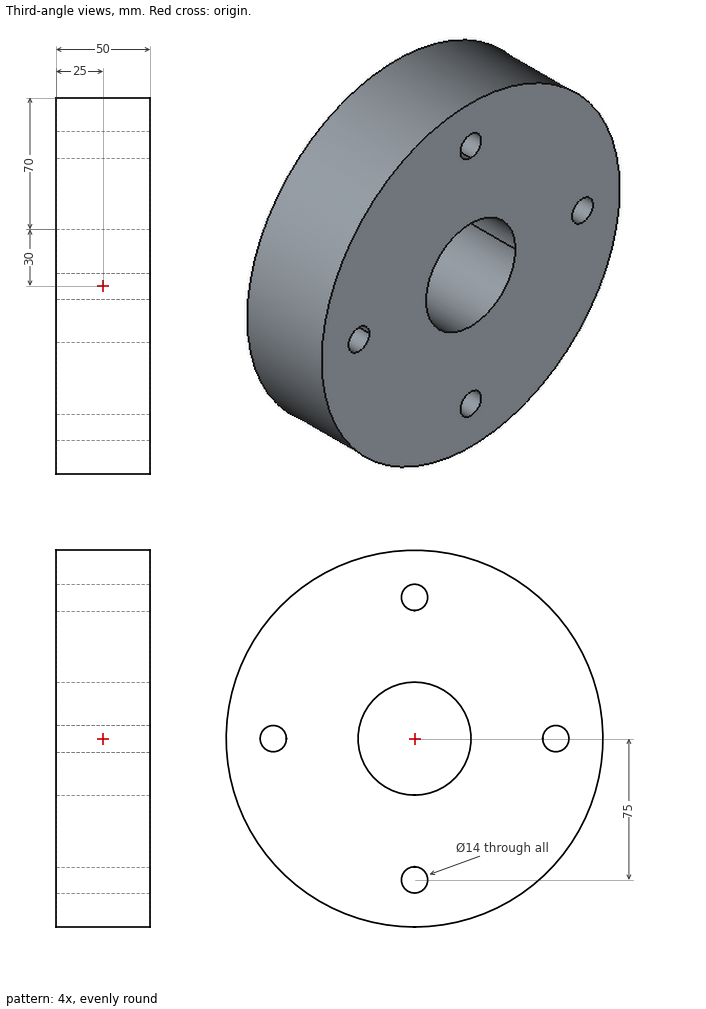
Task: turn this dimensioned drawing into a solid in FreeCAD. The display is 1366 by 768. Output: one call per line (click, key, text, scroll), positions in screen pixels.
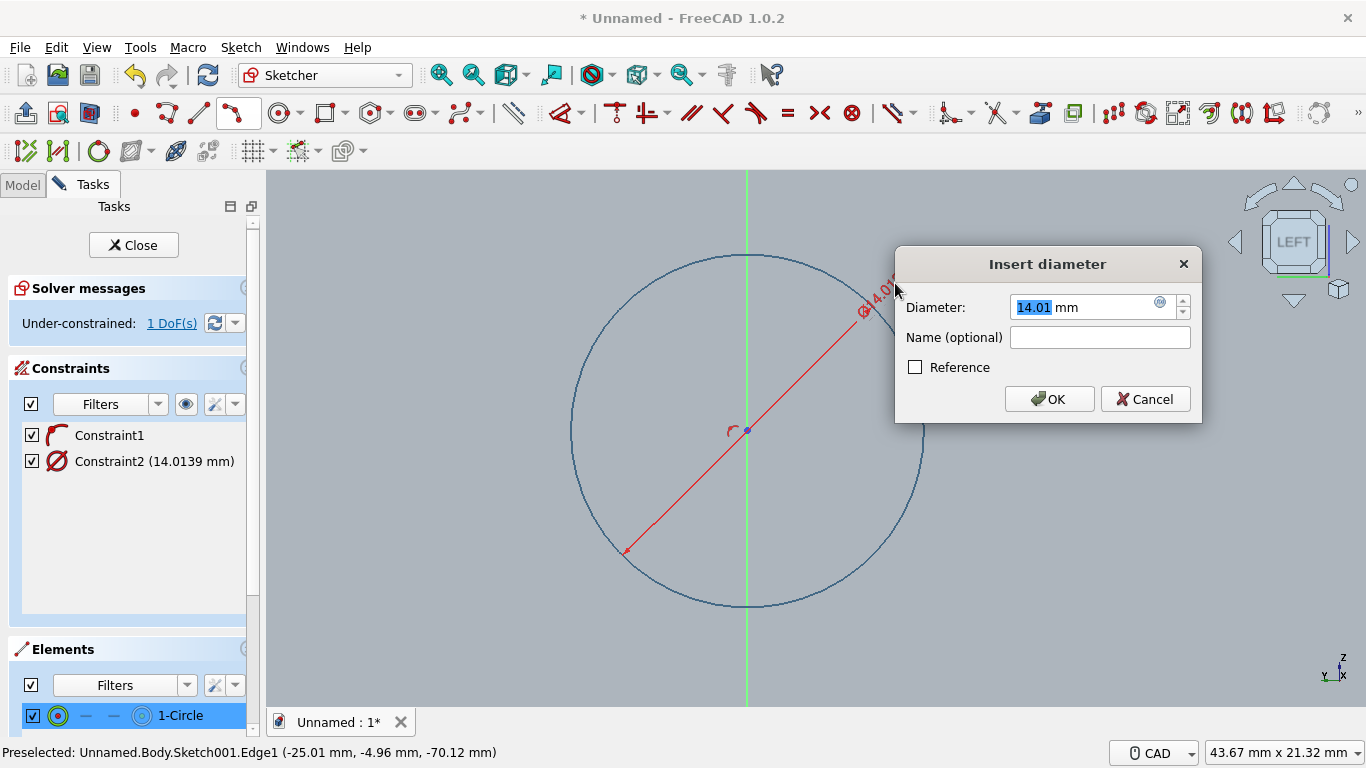
text(14)
key(Return)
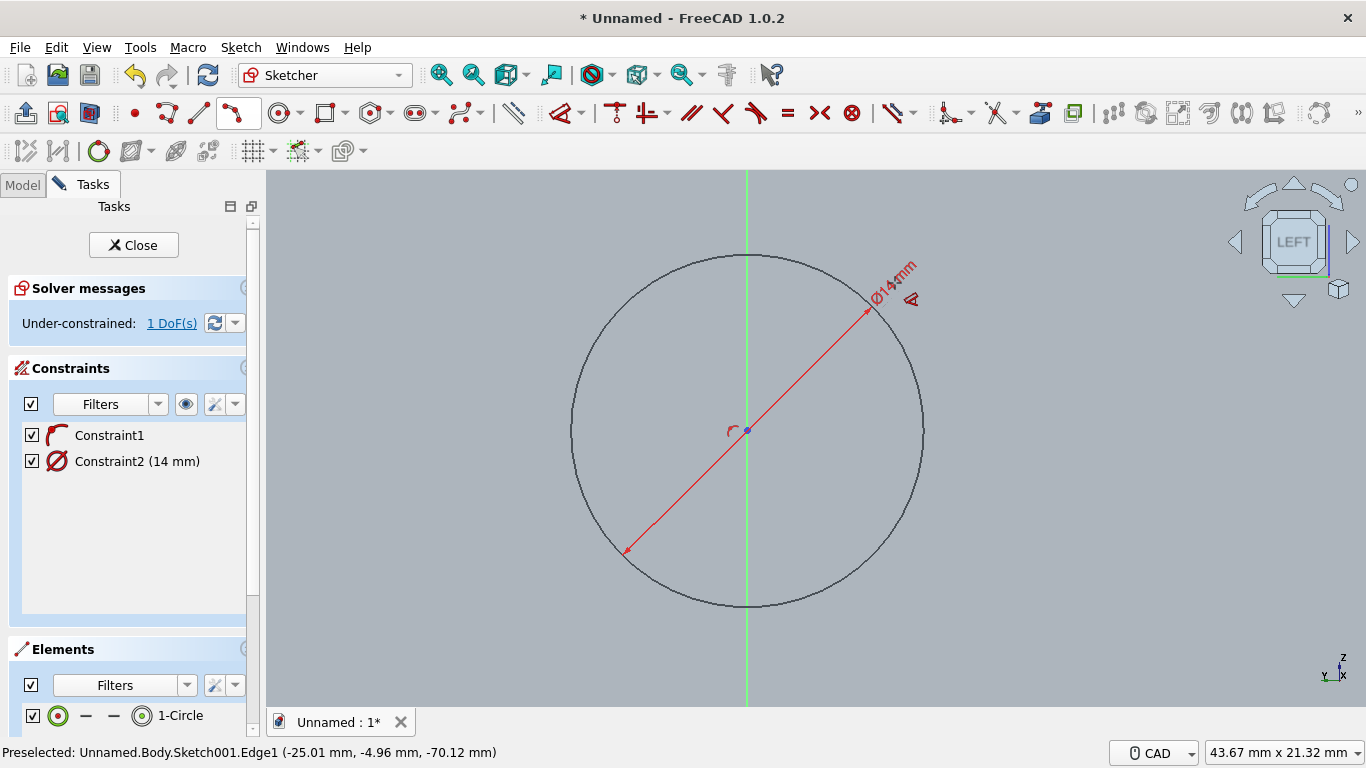
click(747, 431)
click(781, 314)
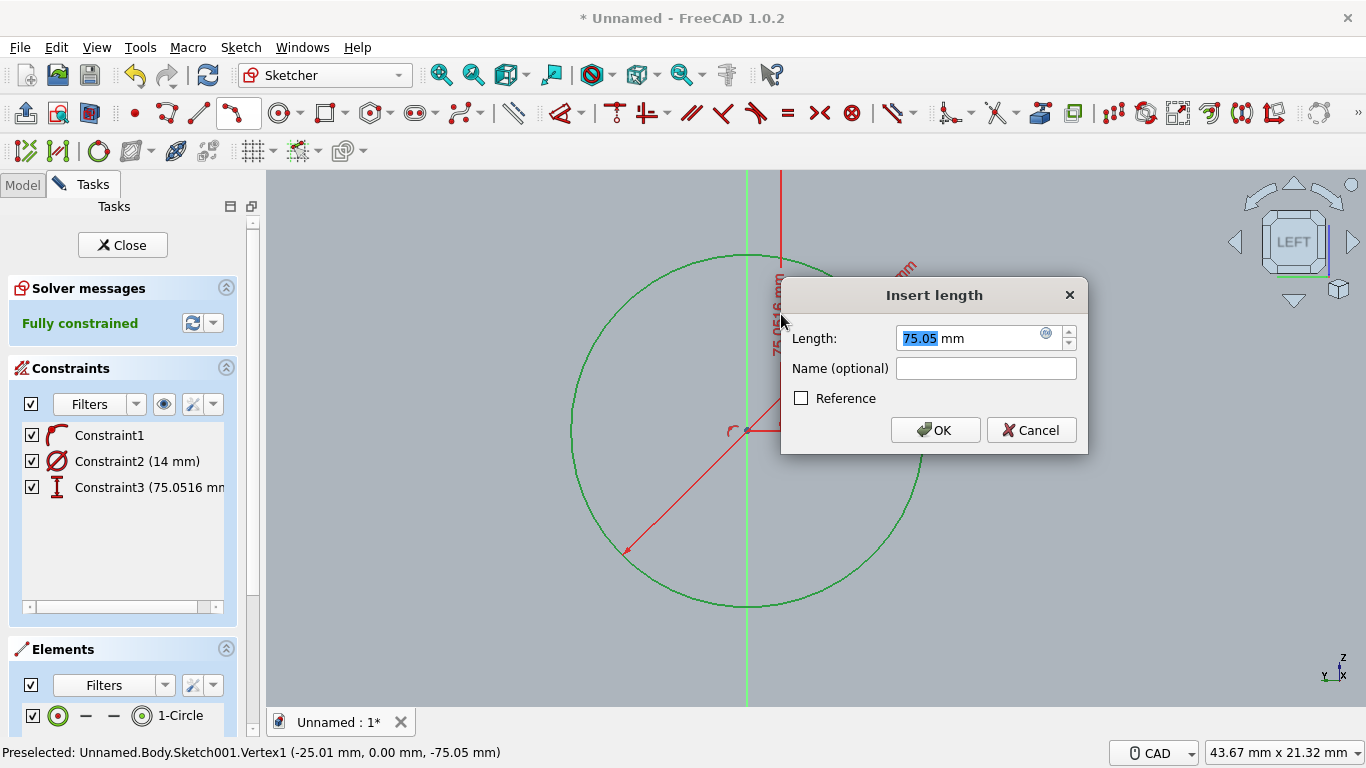
text(75)
key(Return)
key(Escape)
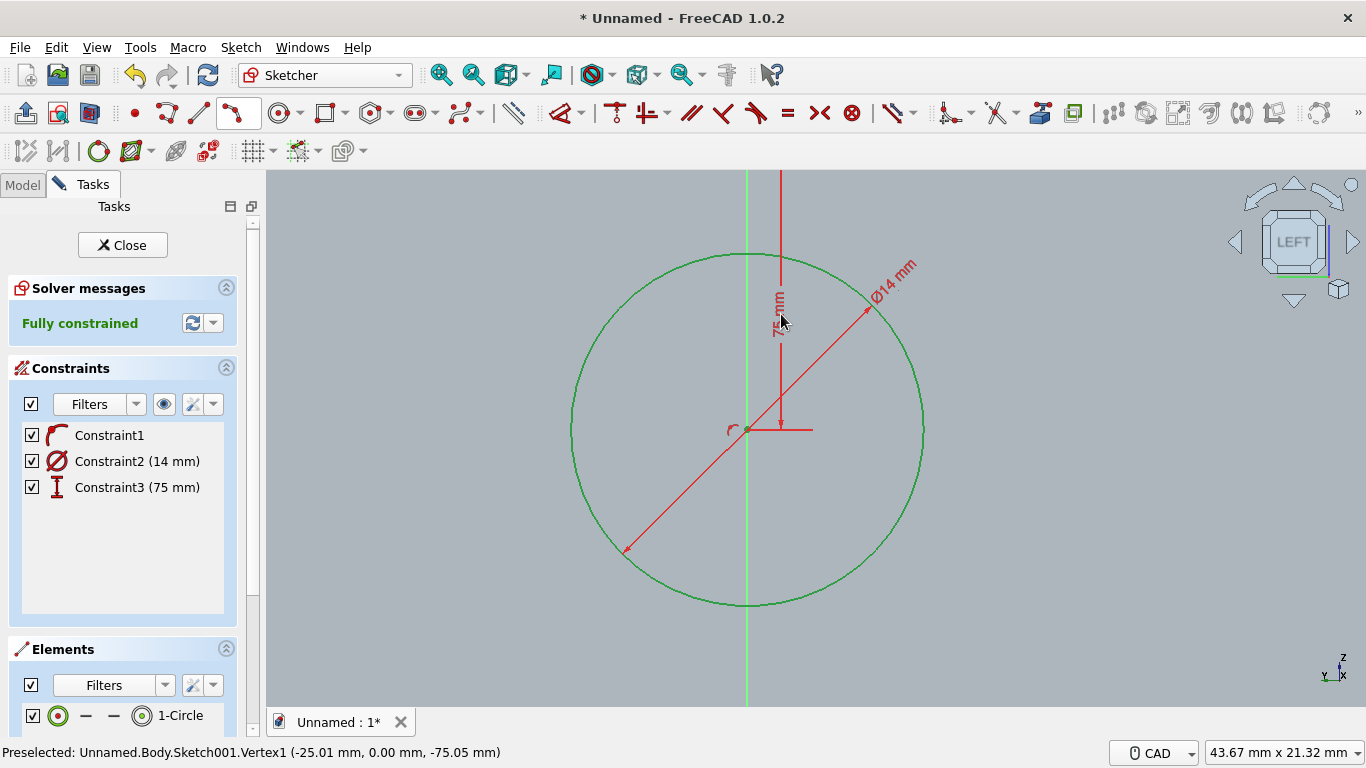
click(123, 245)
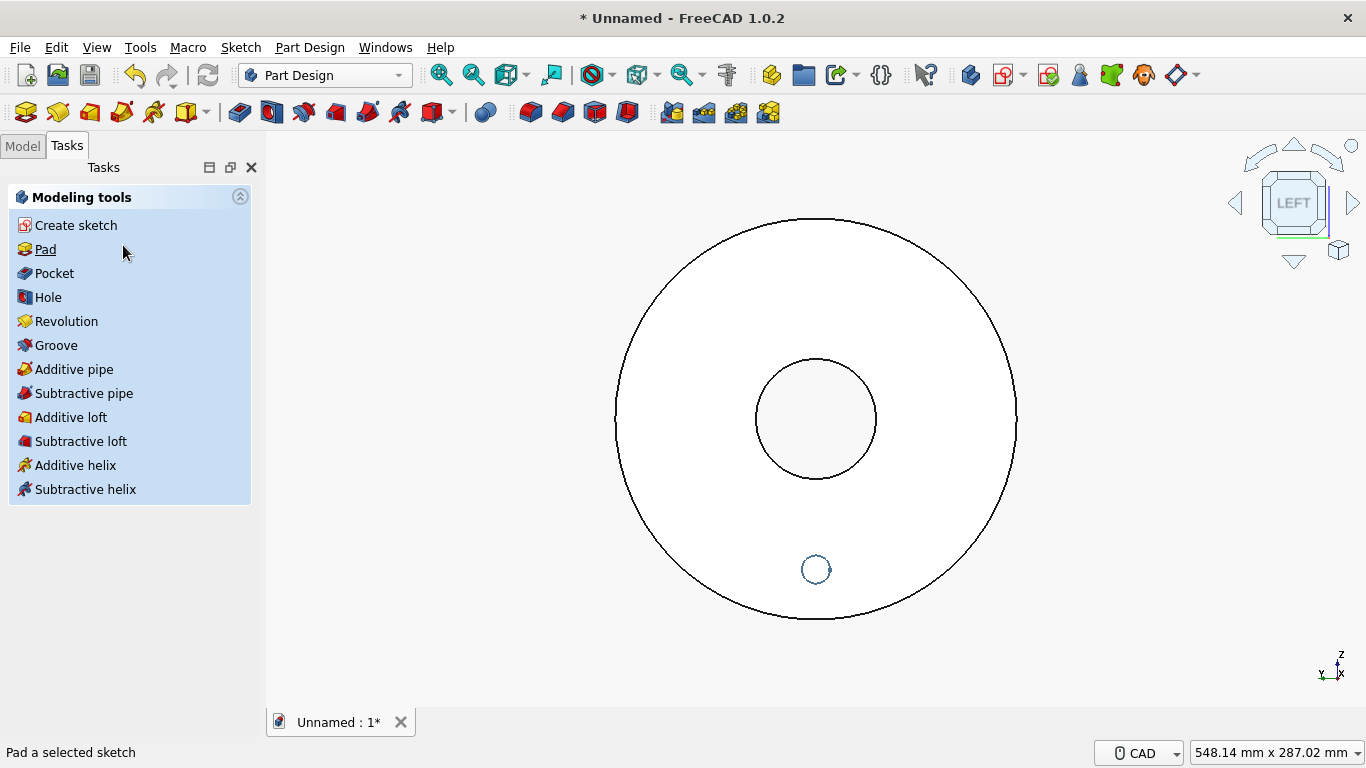
click(272, 112)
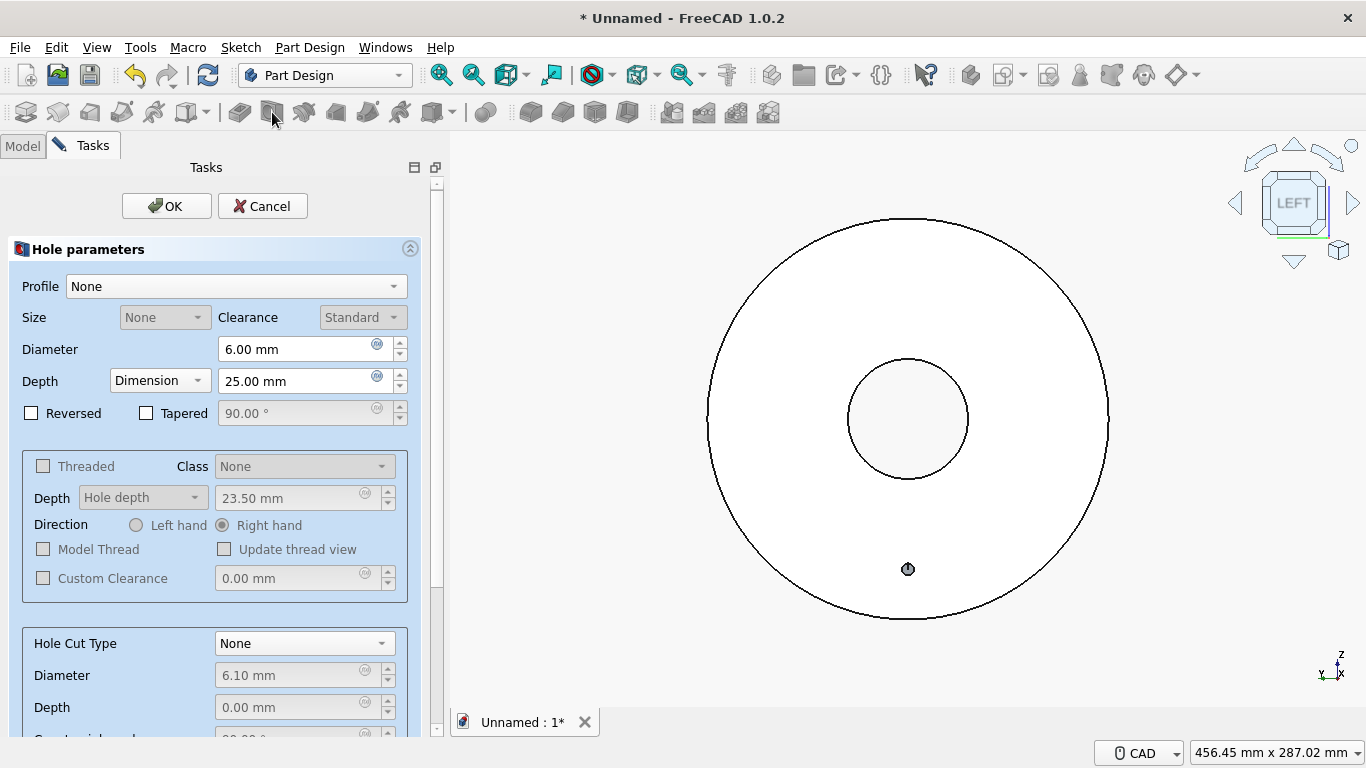
triple_click(305, 349)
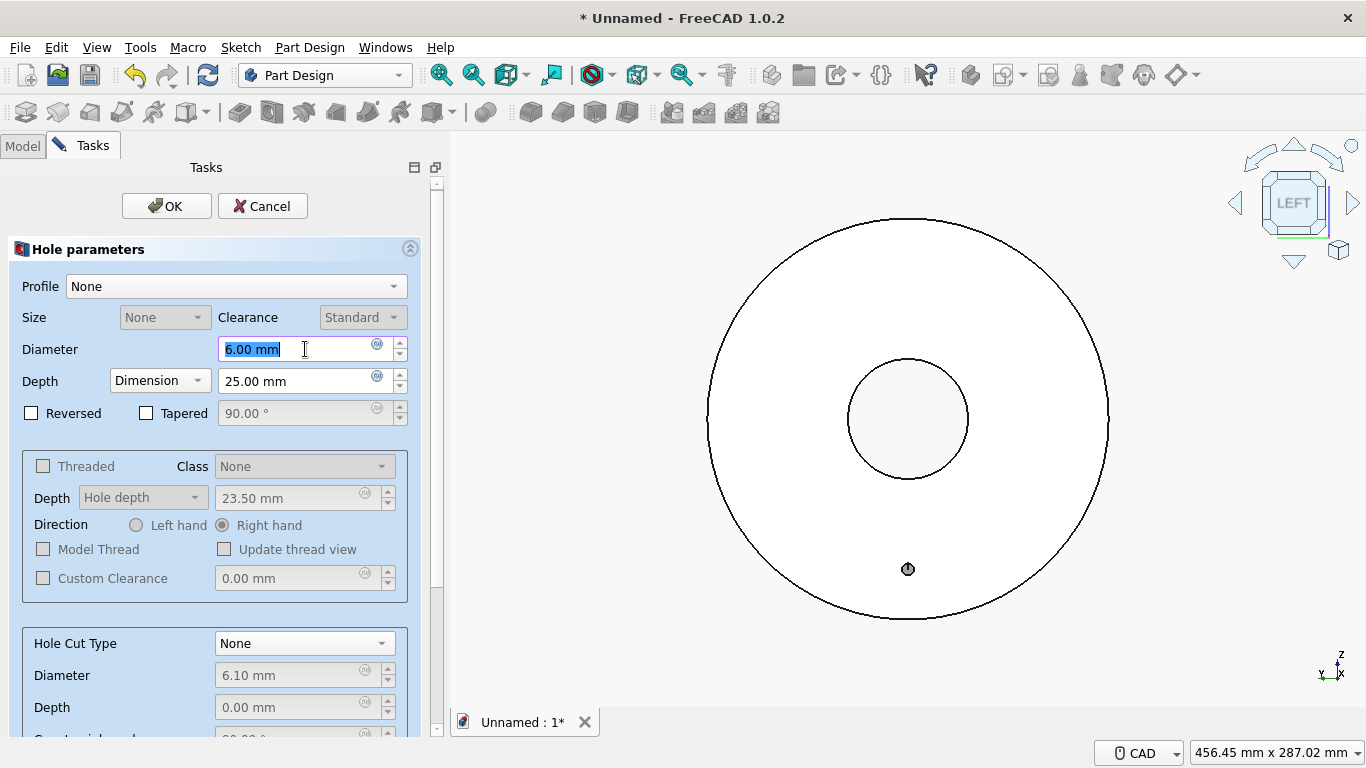
text(14)
key(Tab)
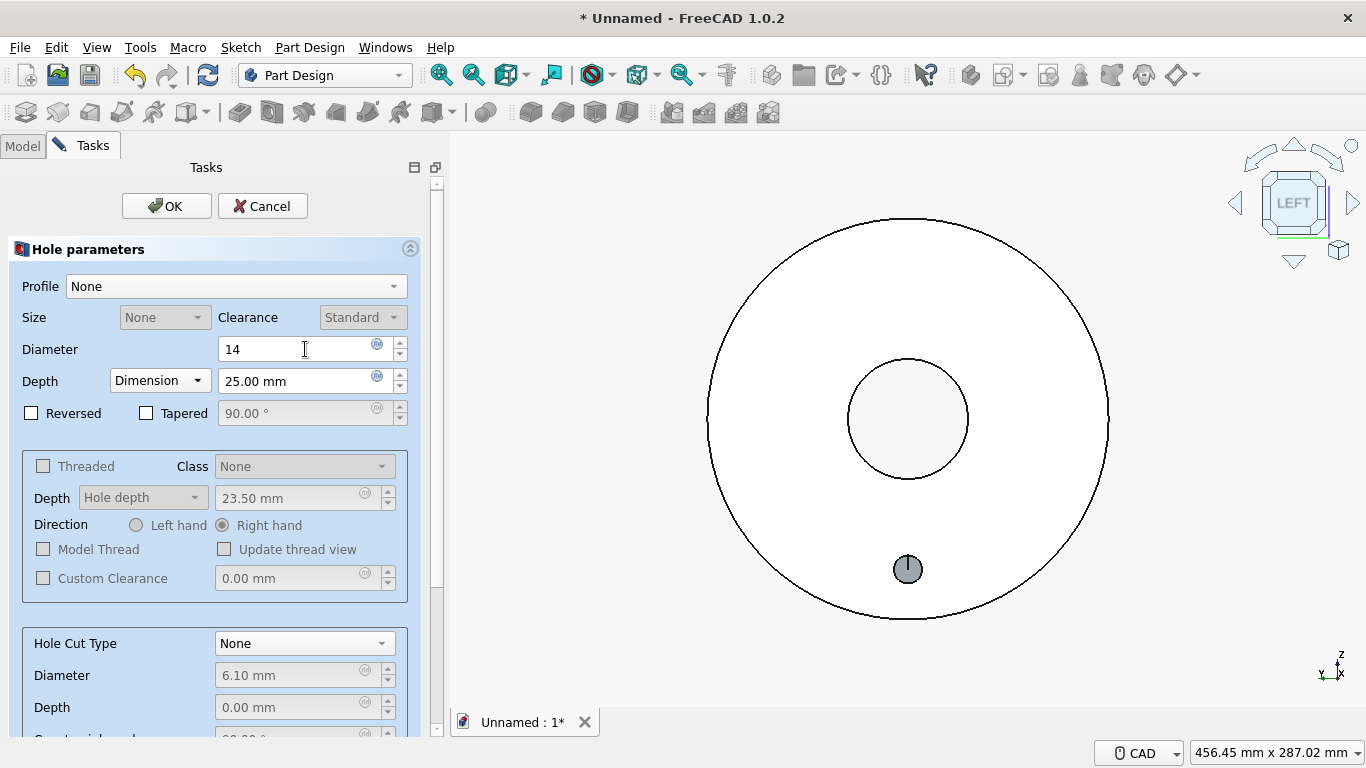
click(161, 380)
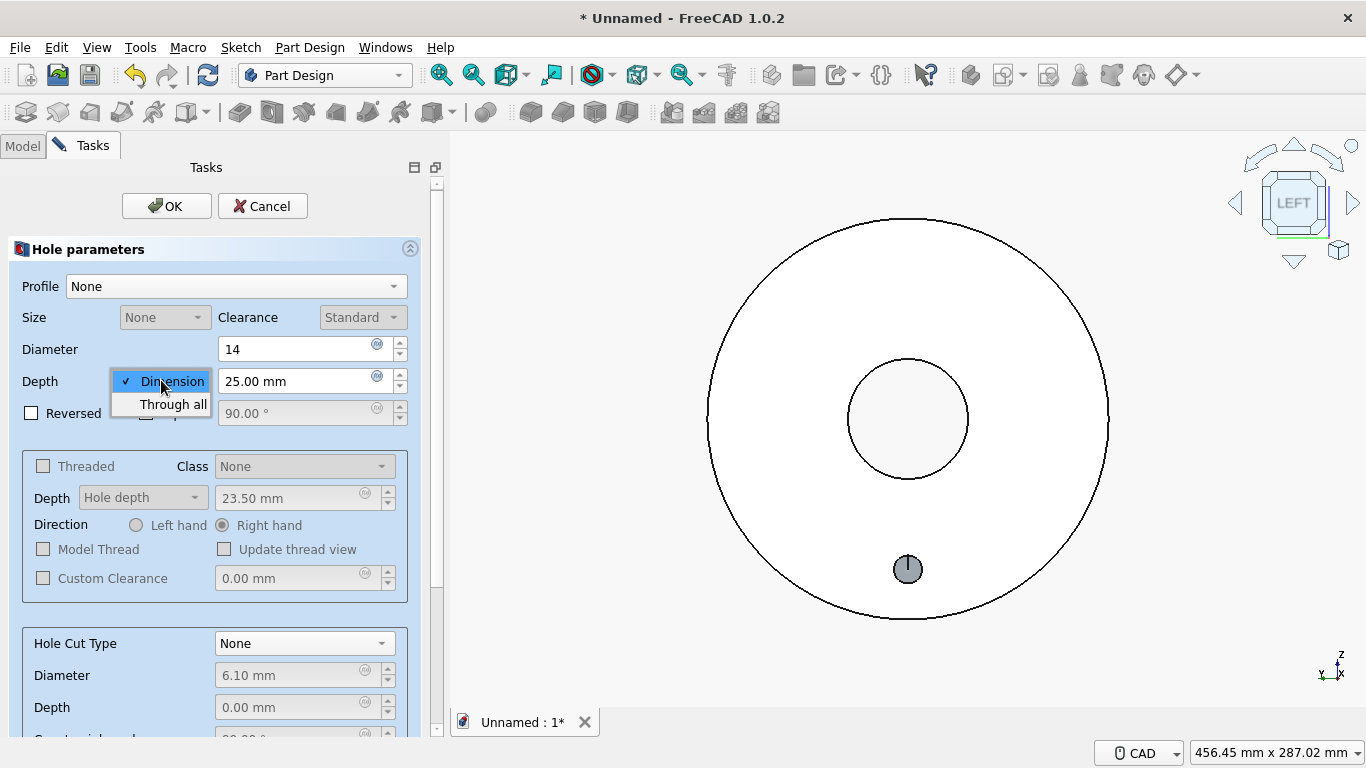
click(160, 404)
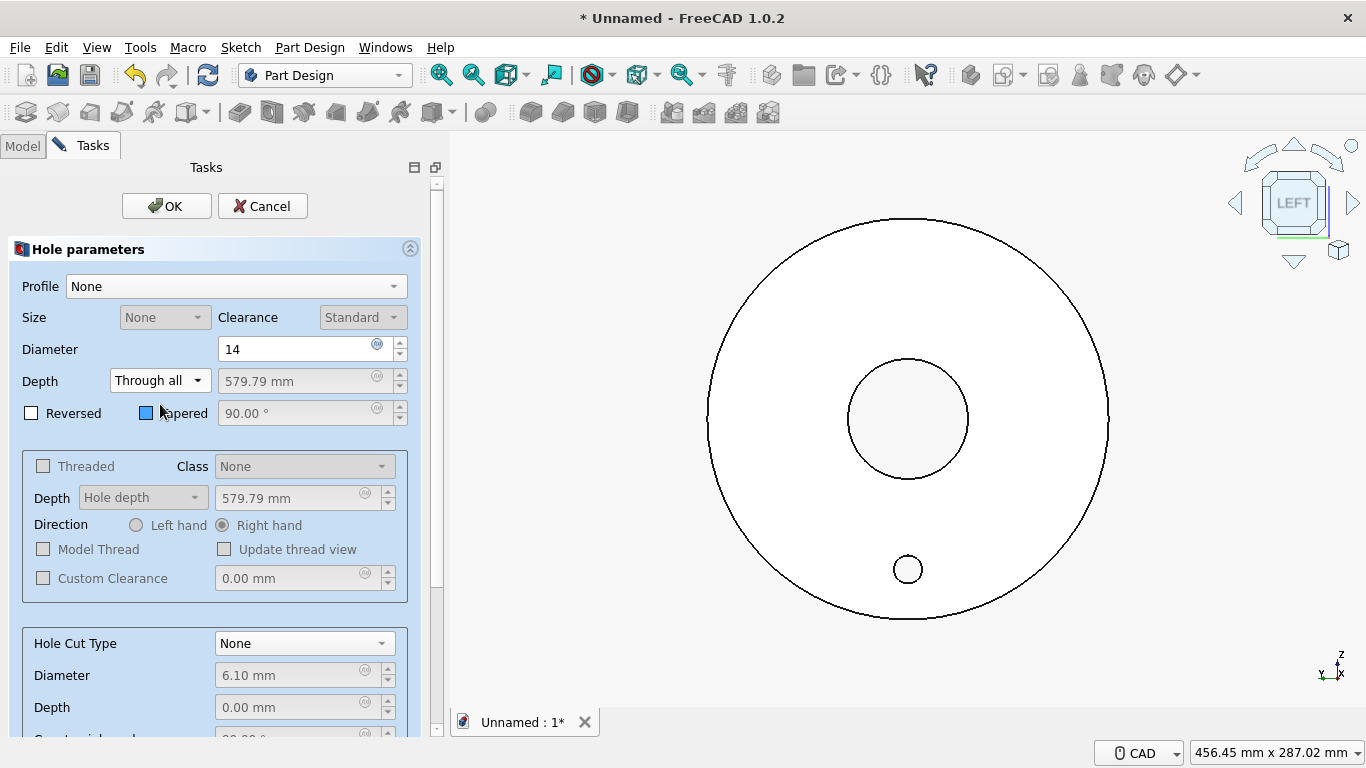
click(167, 206)